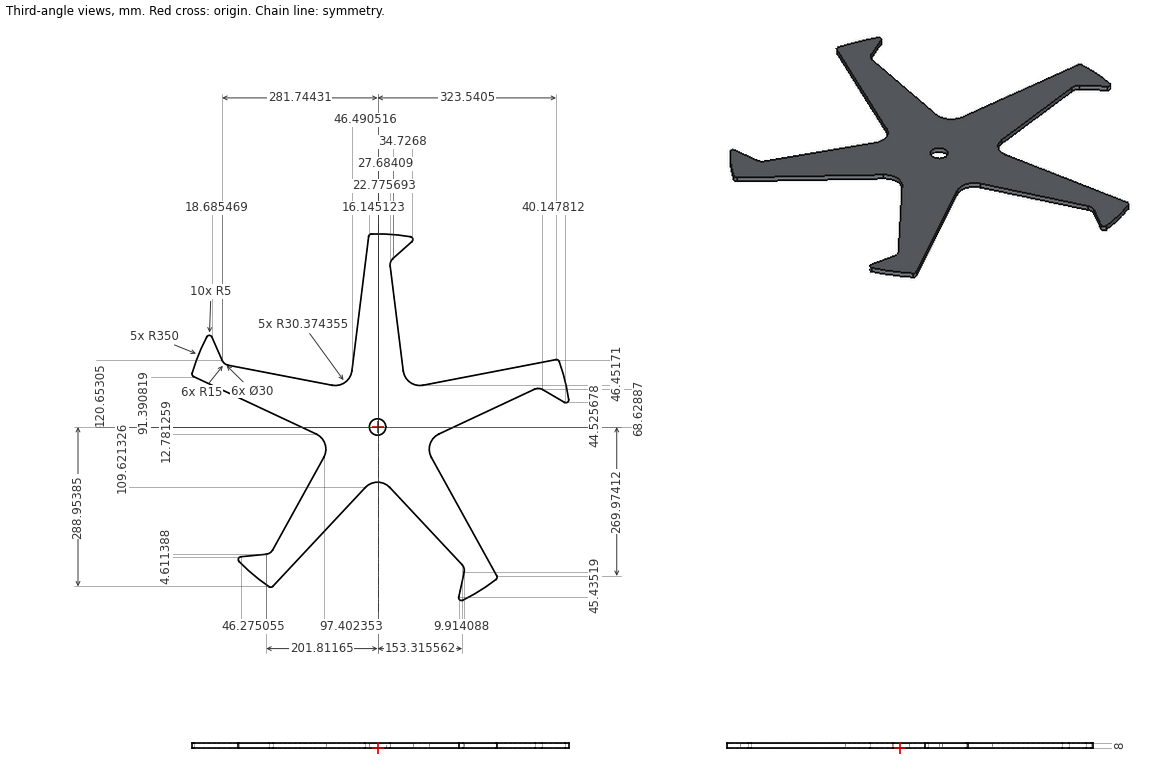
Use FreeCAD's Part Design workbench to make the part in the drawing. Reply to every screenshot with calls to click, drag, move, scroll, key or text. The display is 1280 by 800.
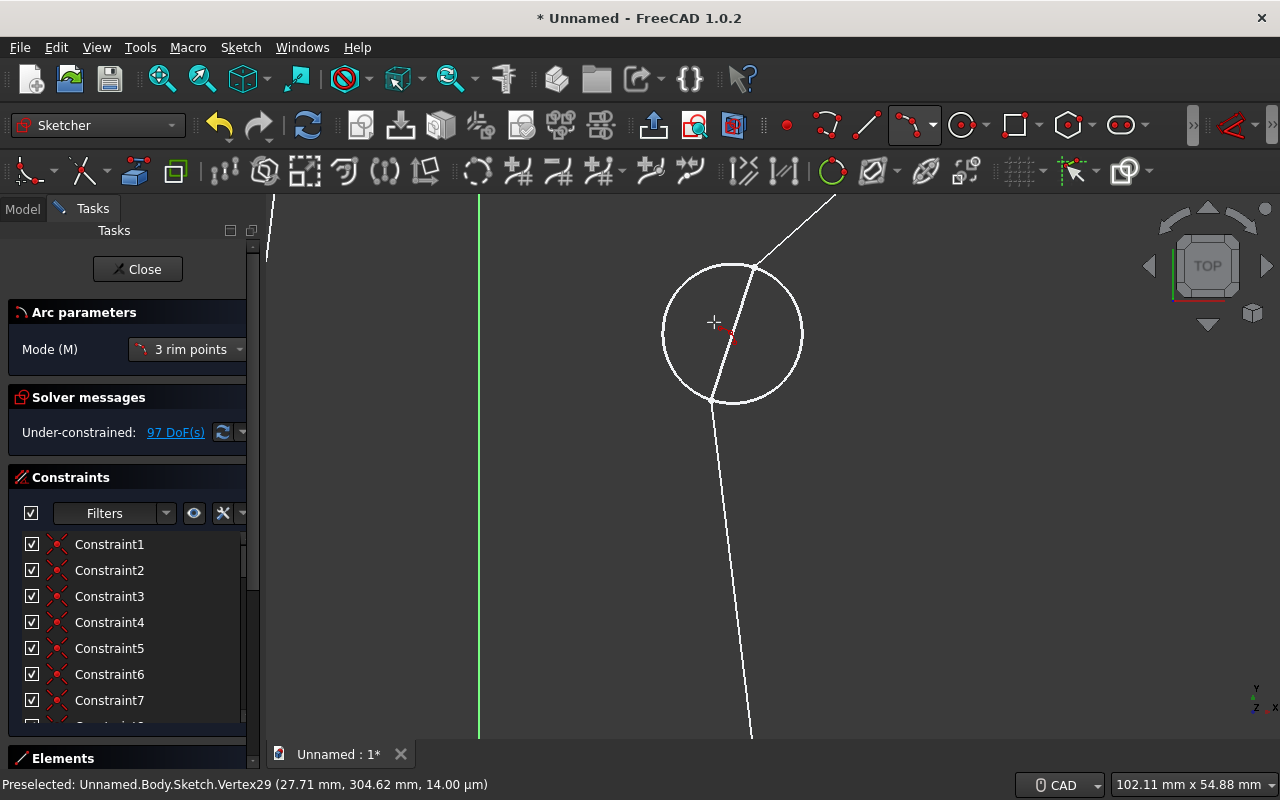
click(713, 320)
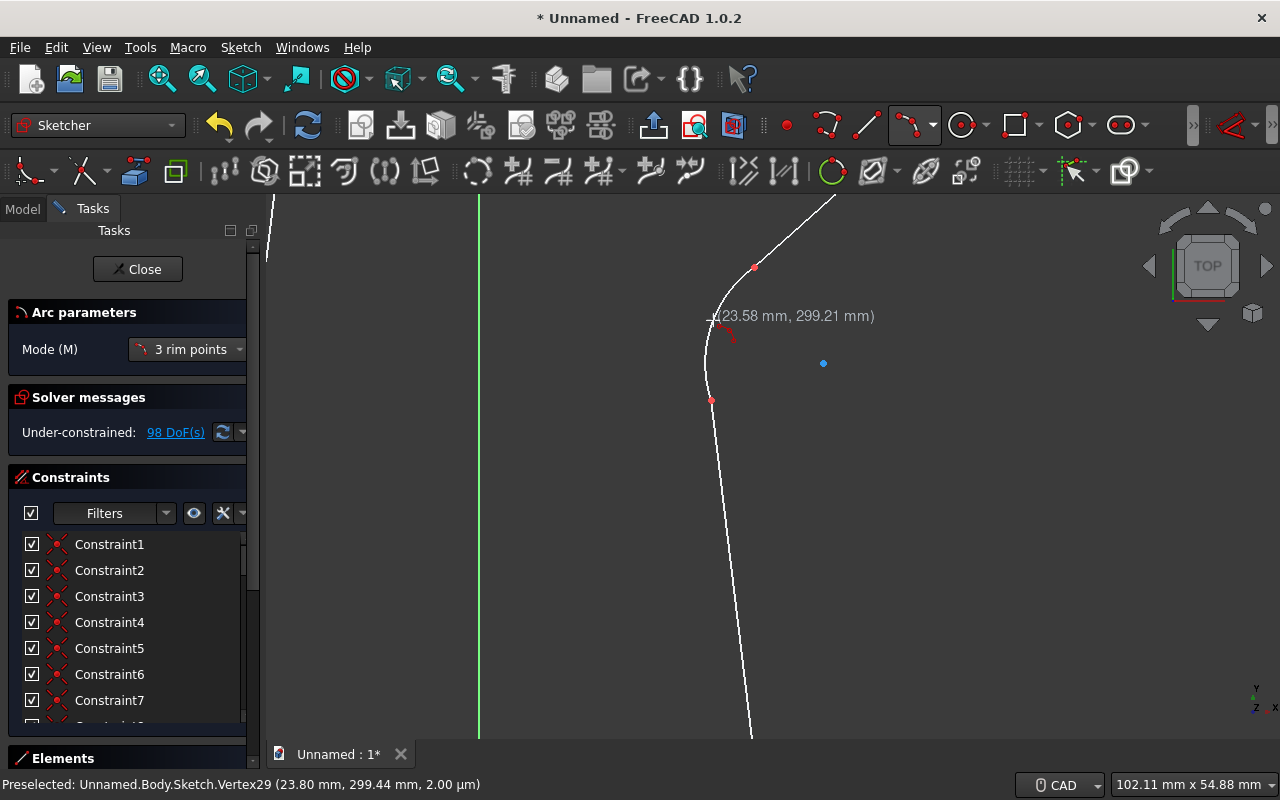
scroll(714, 328, down, 15)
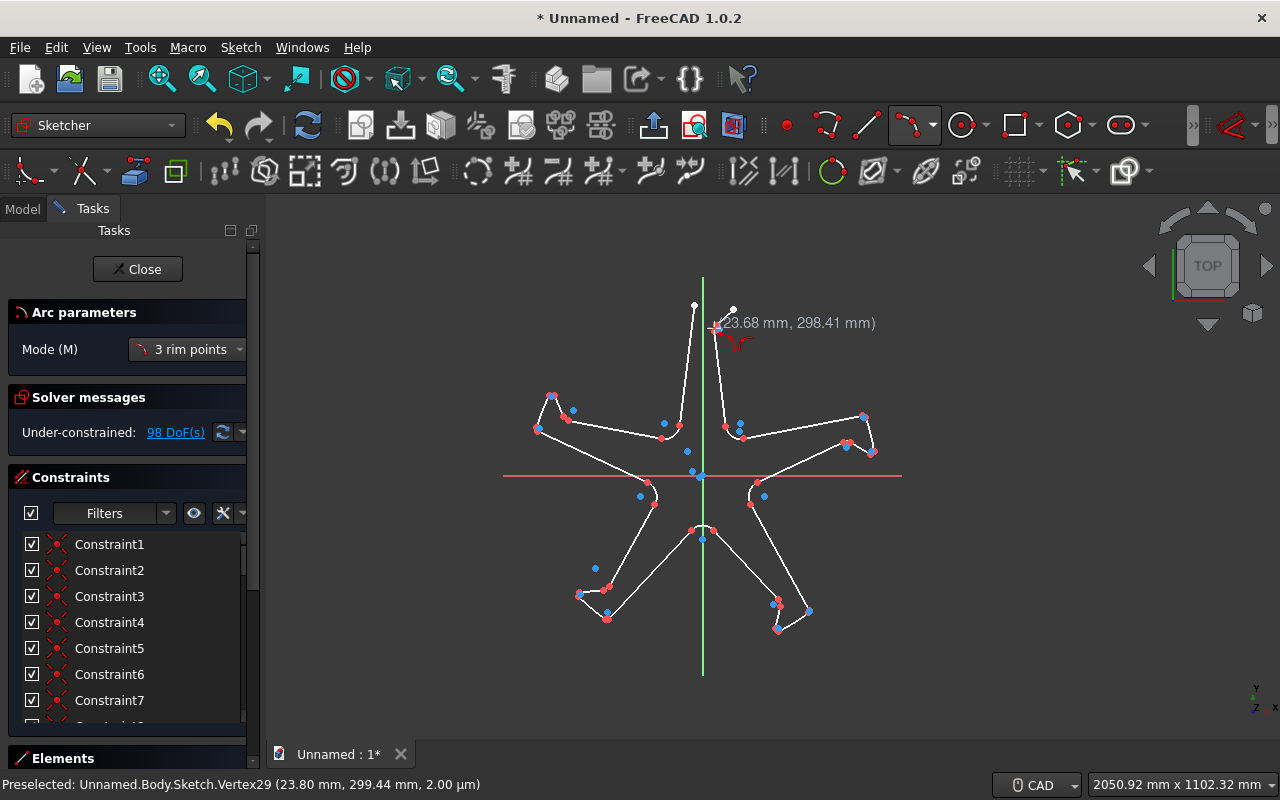
scroll(734, 310, up, 2)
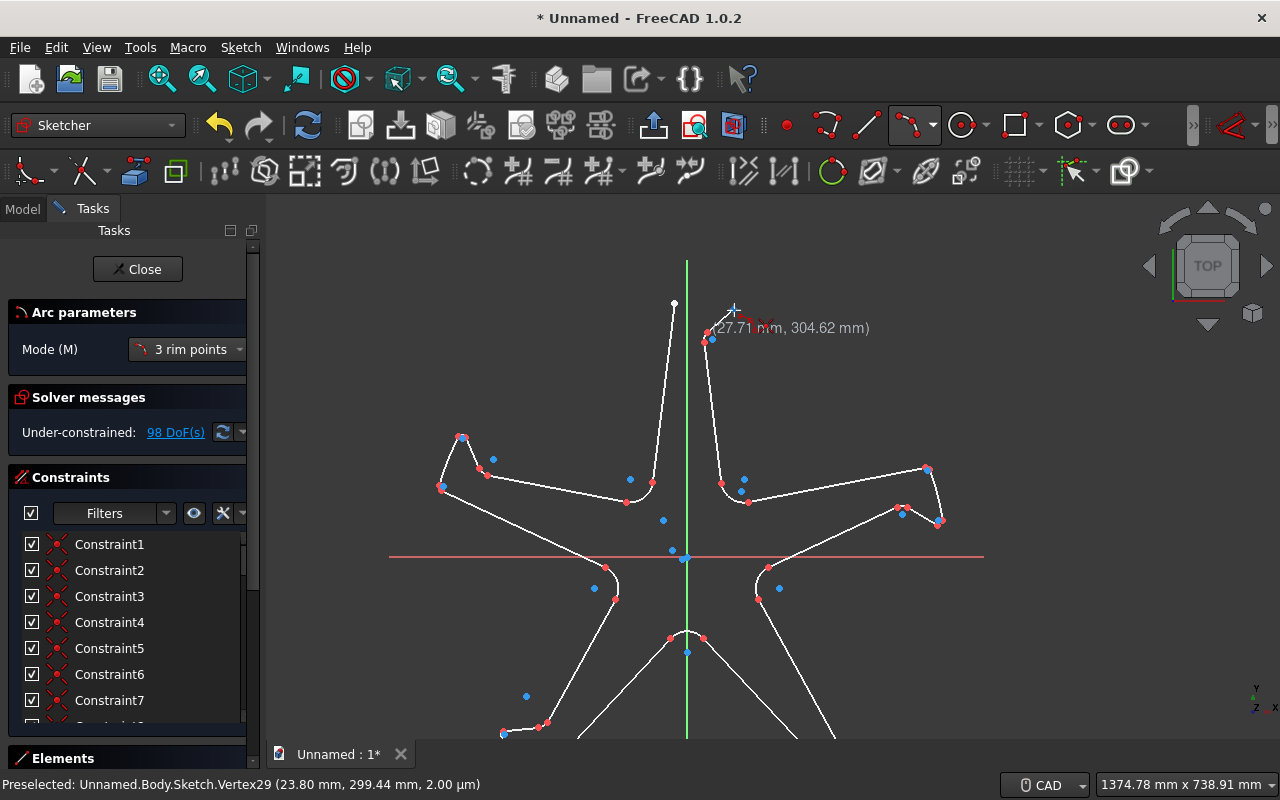
click(733, 310)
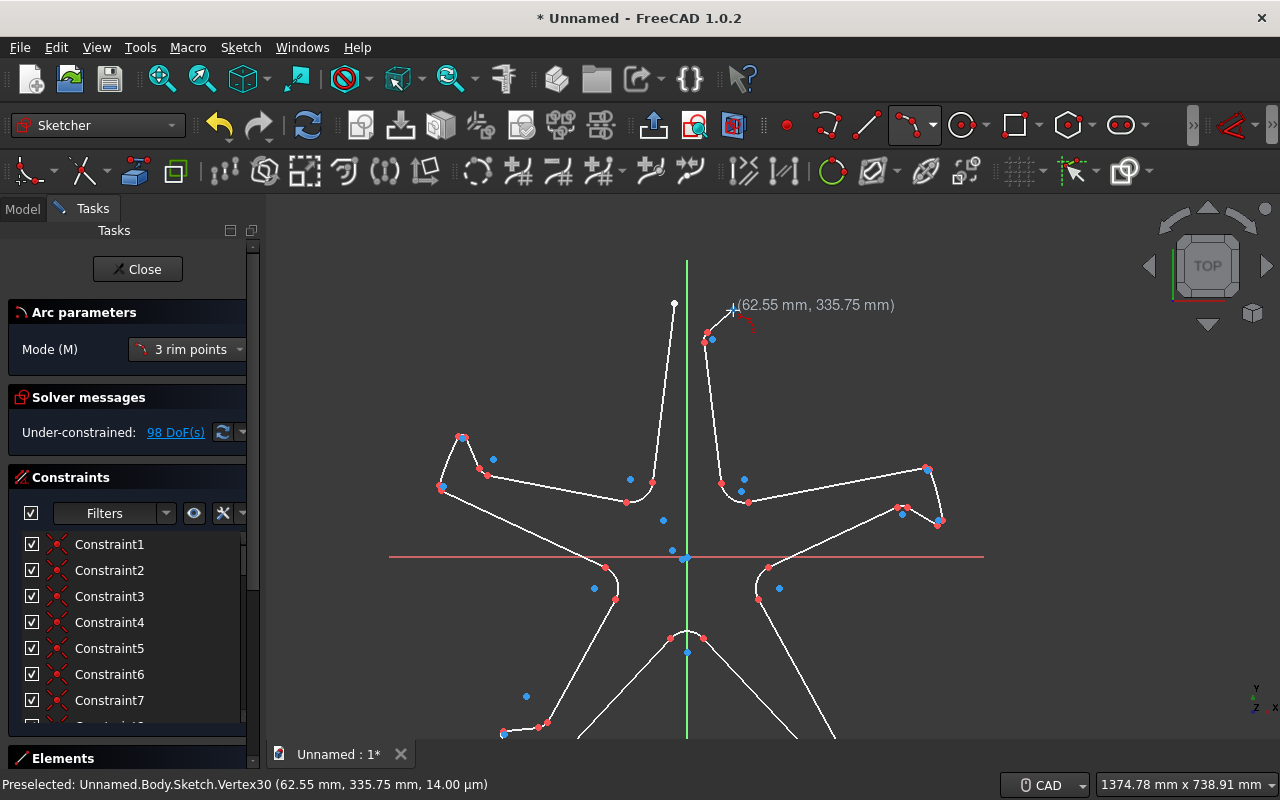
scroll(731, 303, up, 5)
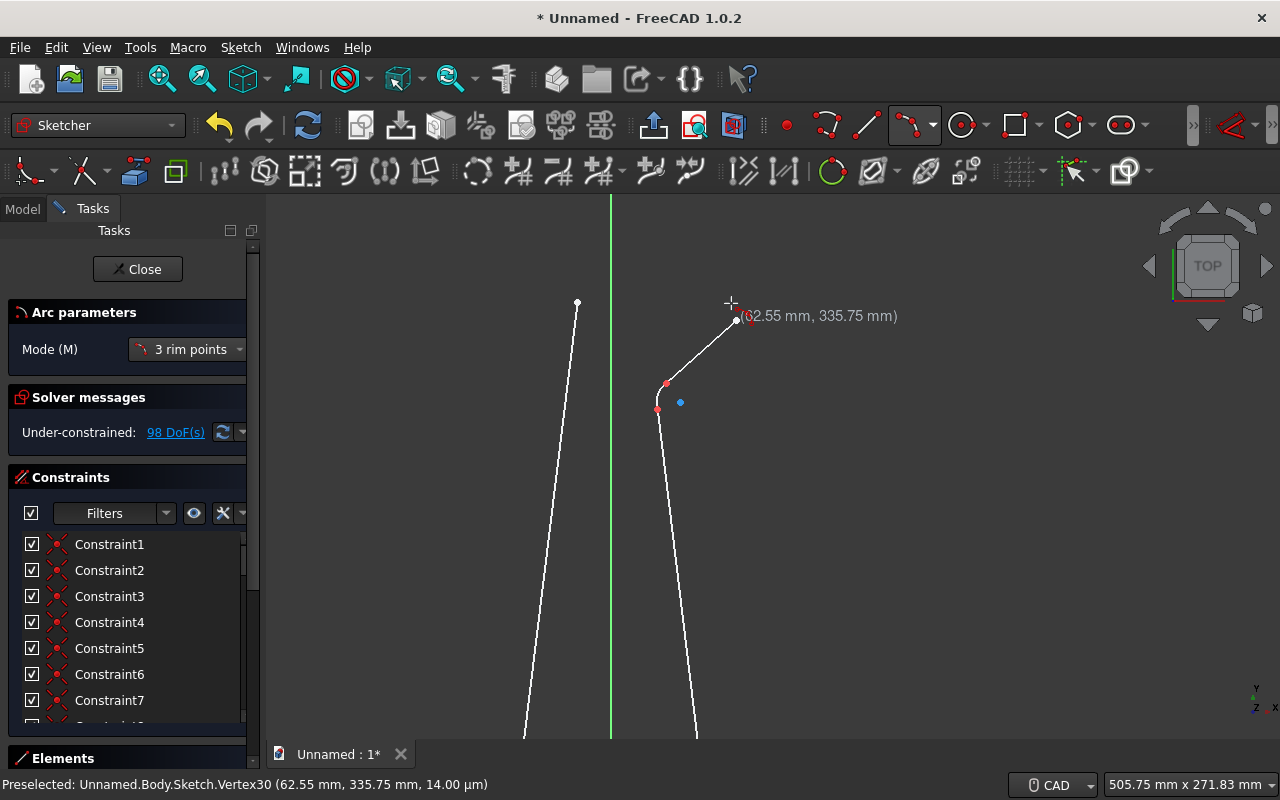
click(731, 302)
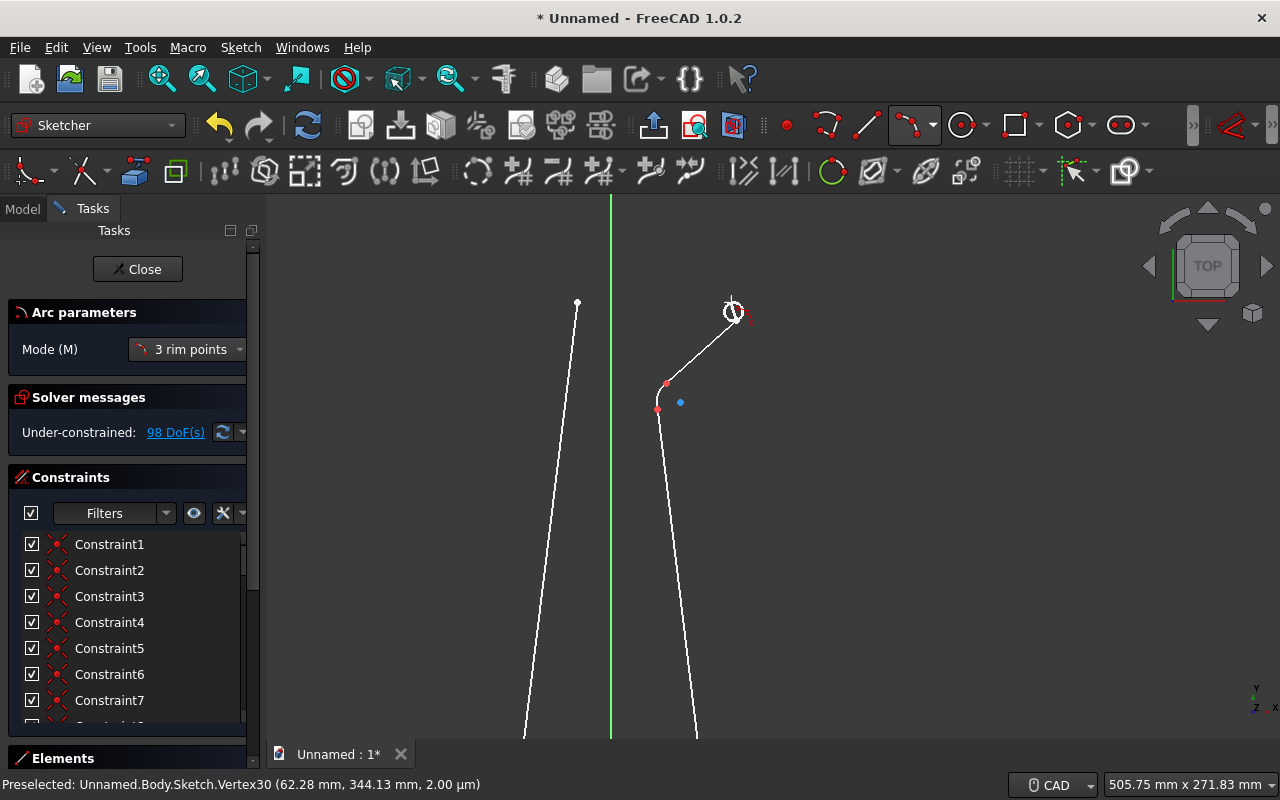
scroll(739, 310, up, 6)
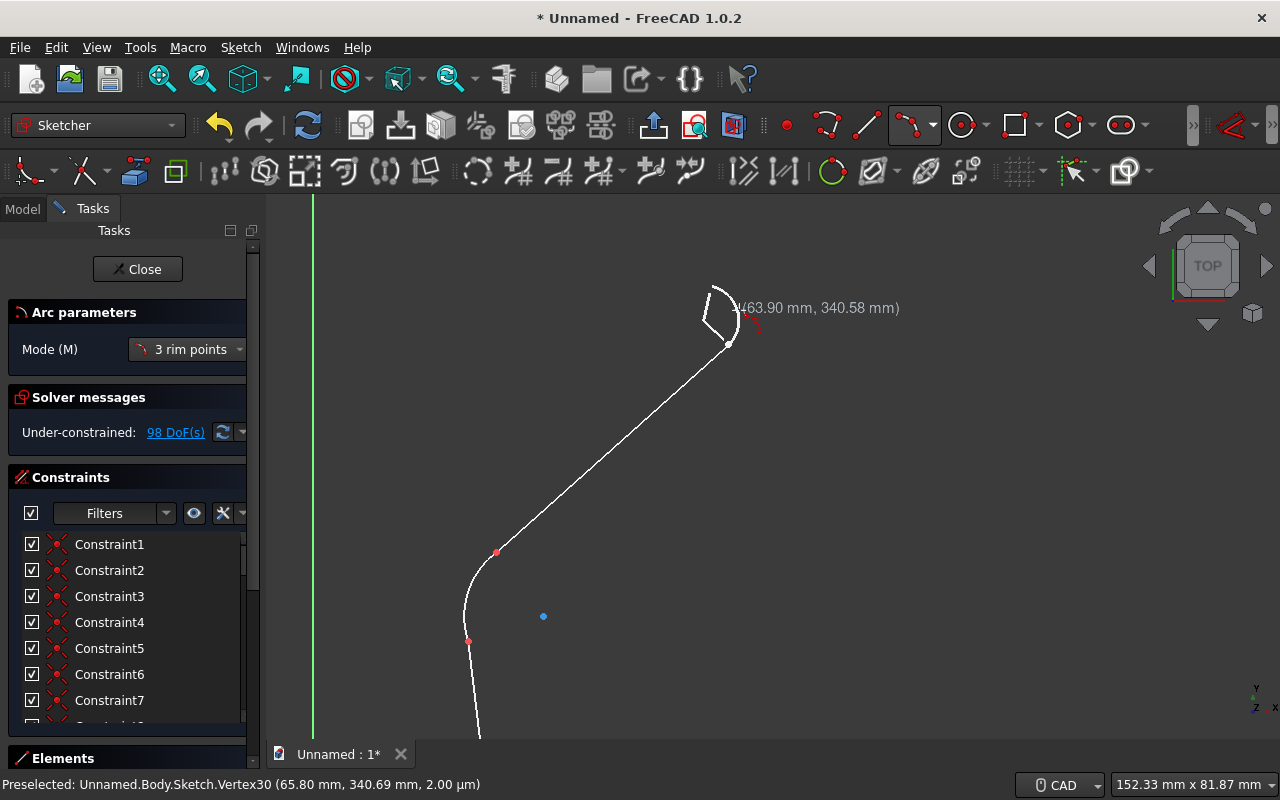
click(738, 308)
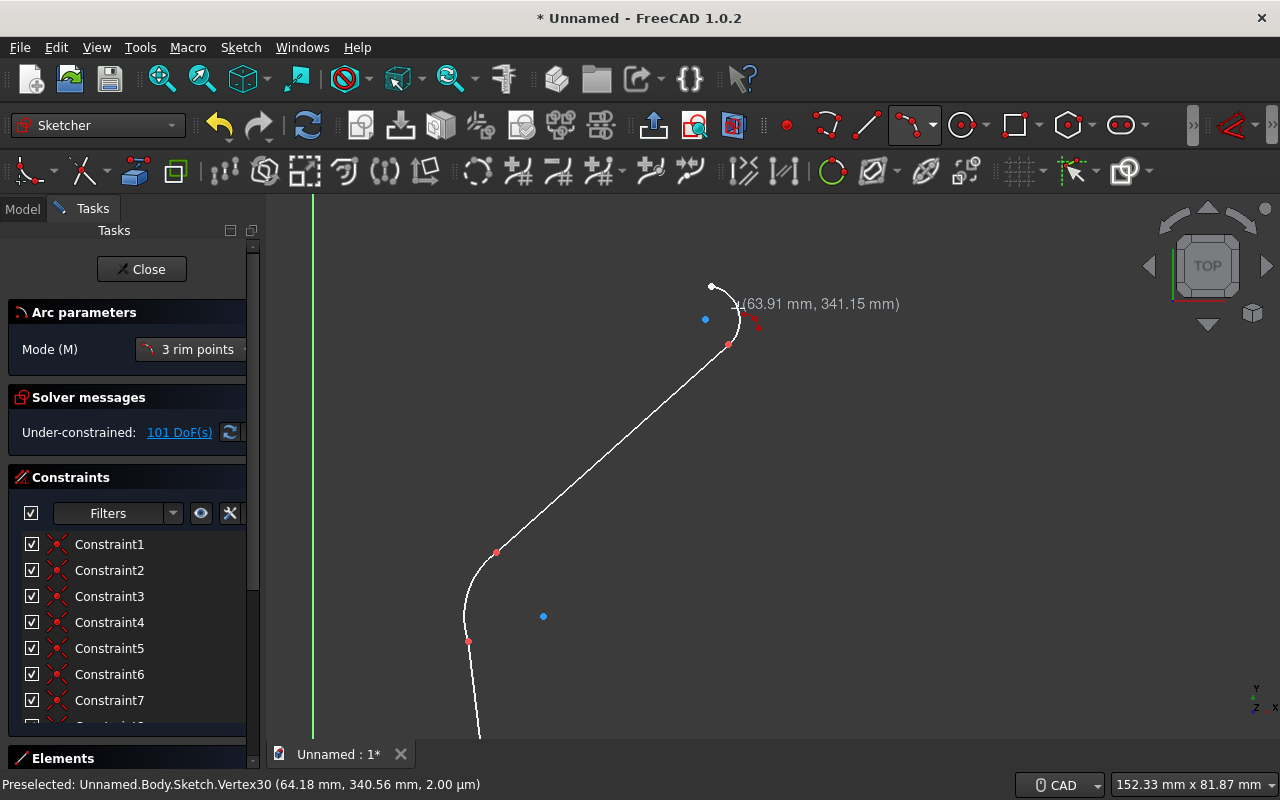
click(711, 286)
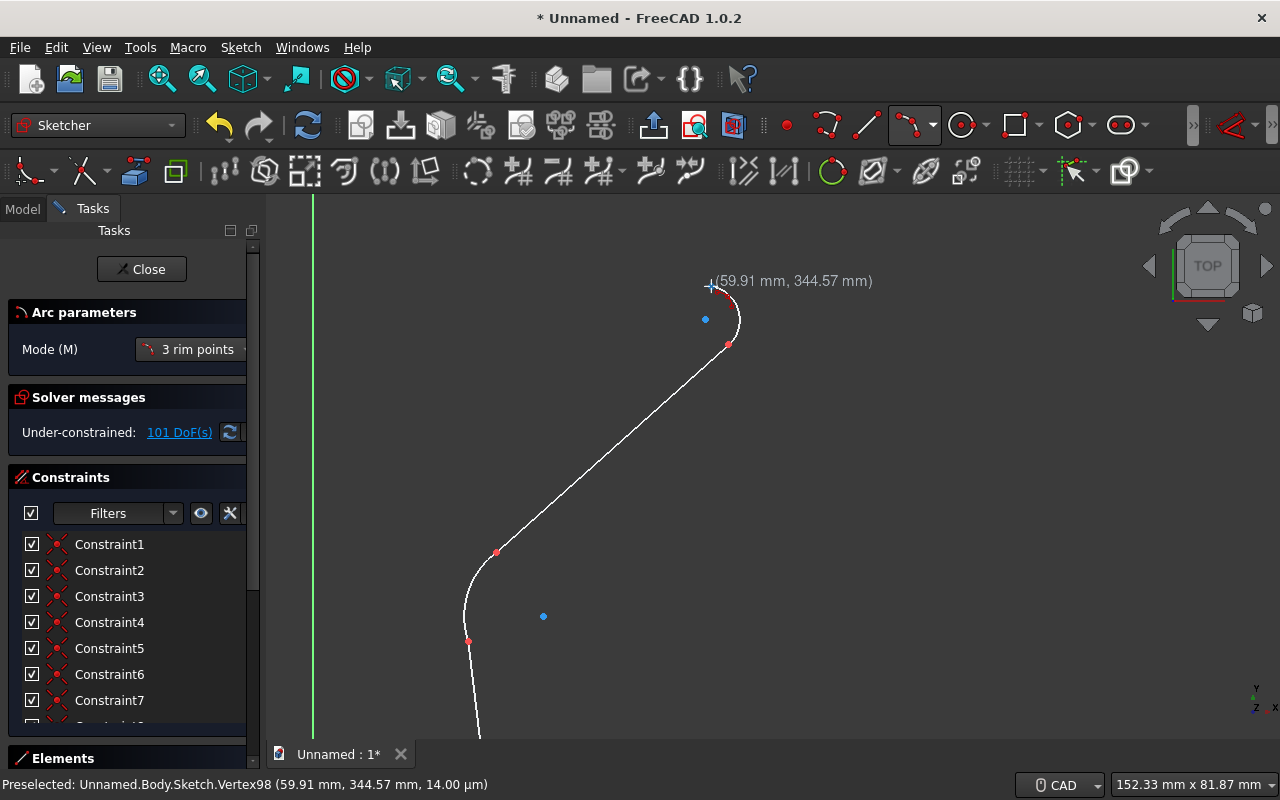
scroll(733, 306, down, 13)